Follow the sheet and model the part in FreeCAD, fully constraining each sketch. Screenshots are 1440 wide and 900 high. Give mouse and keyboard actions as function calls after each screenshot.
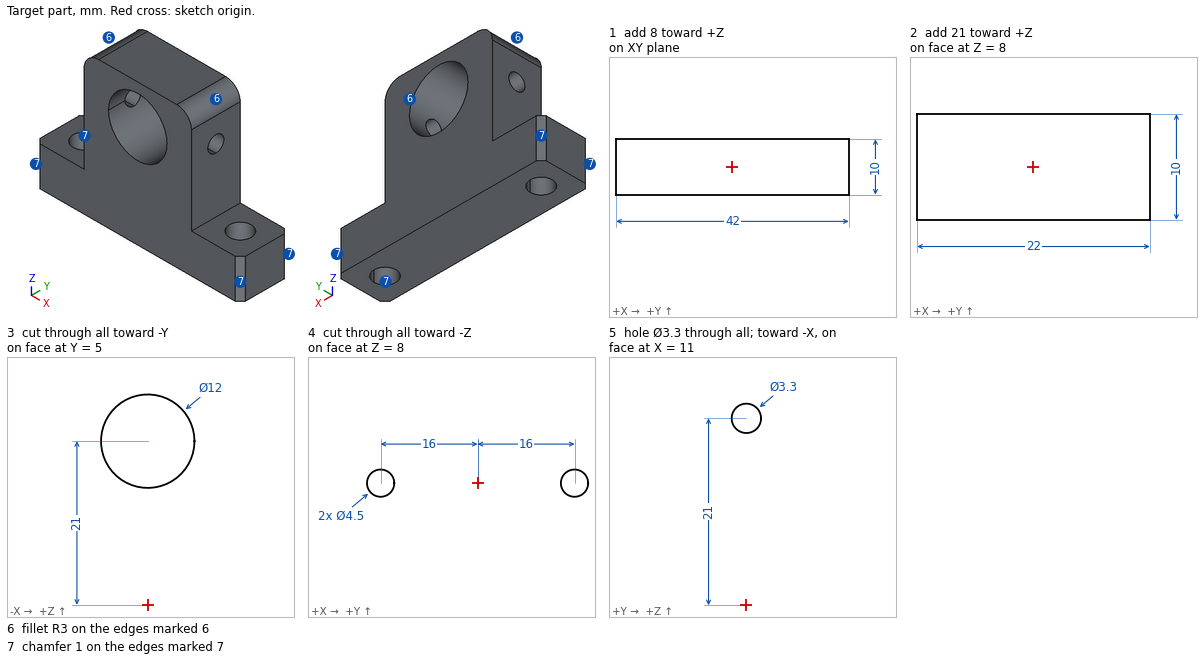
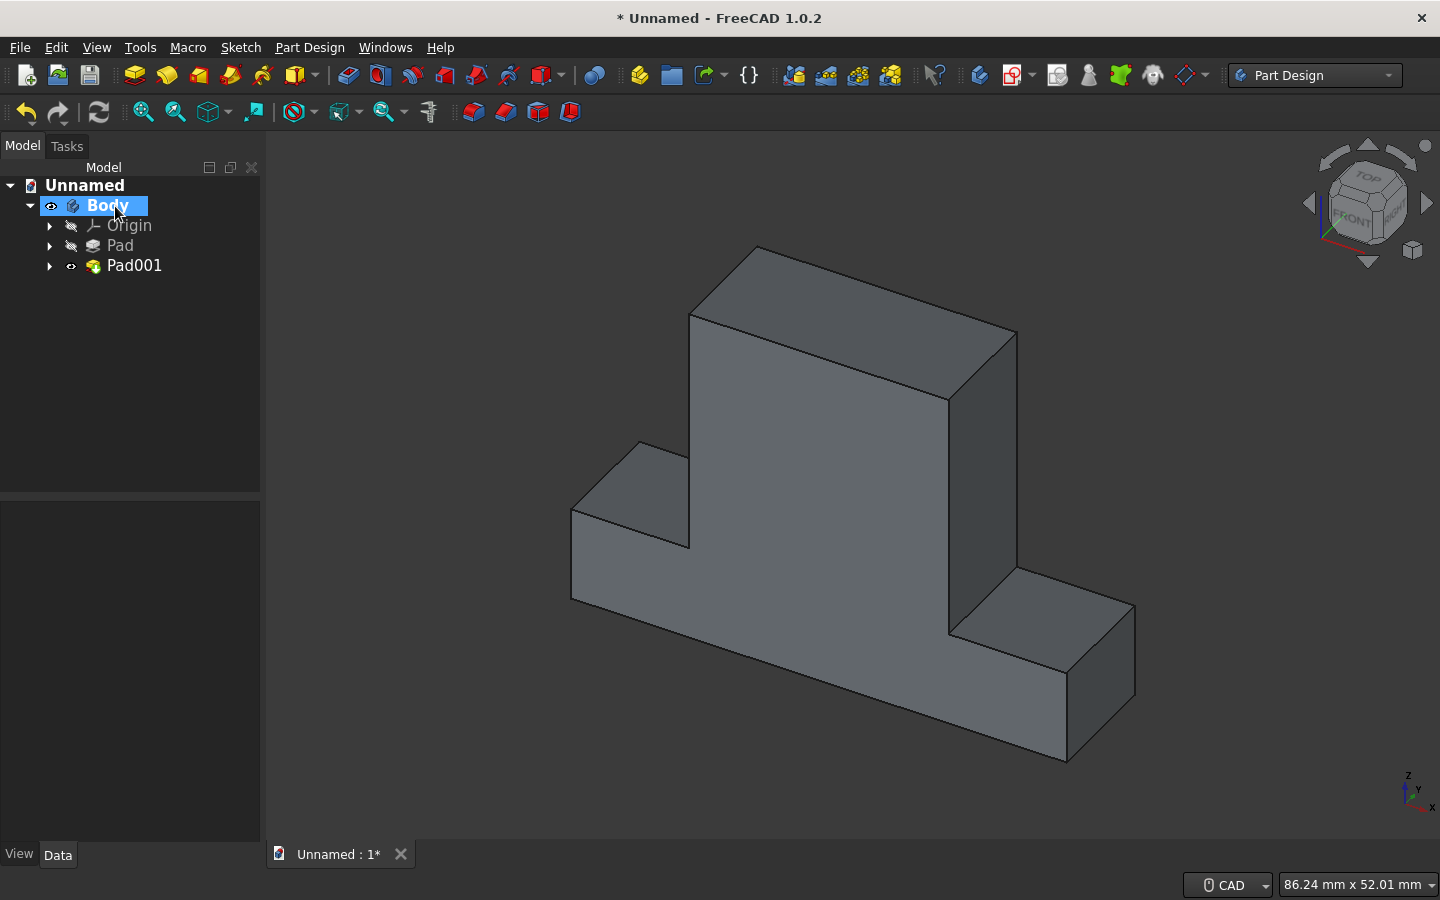
key(4)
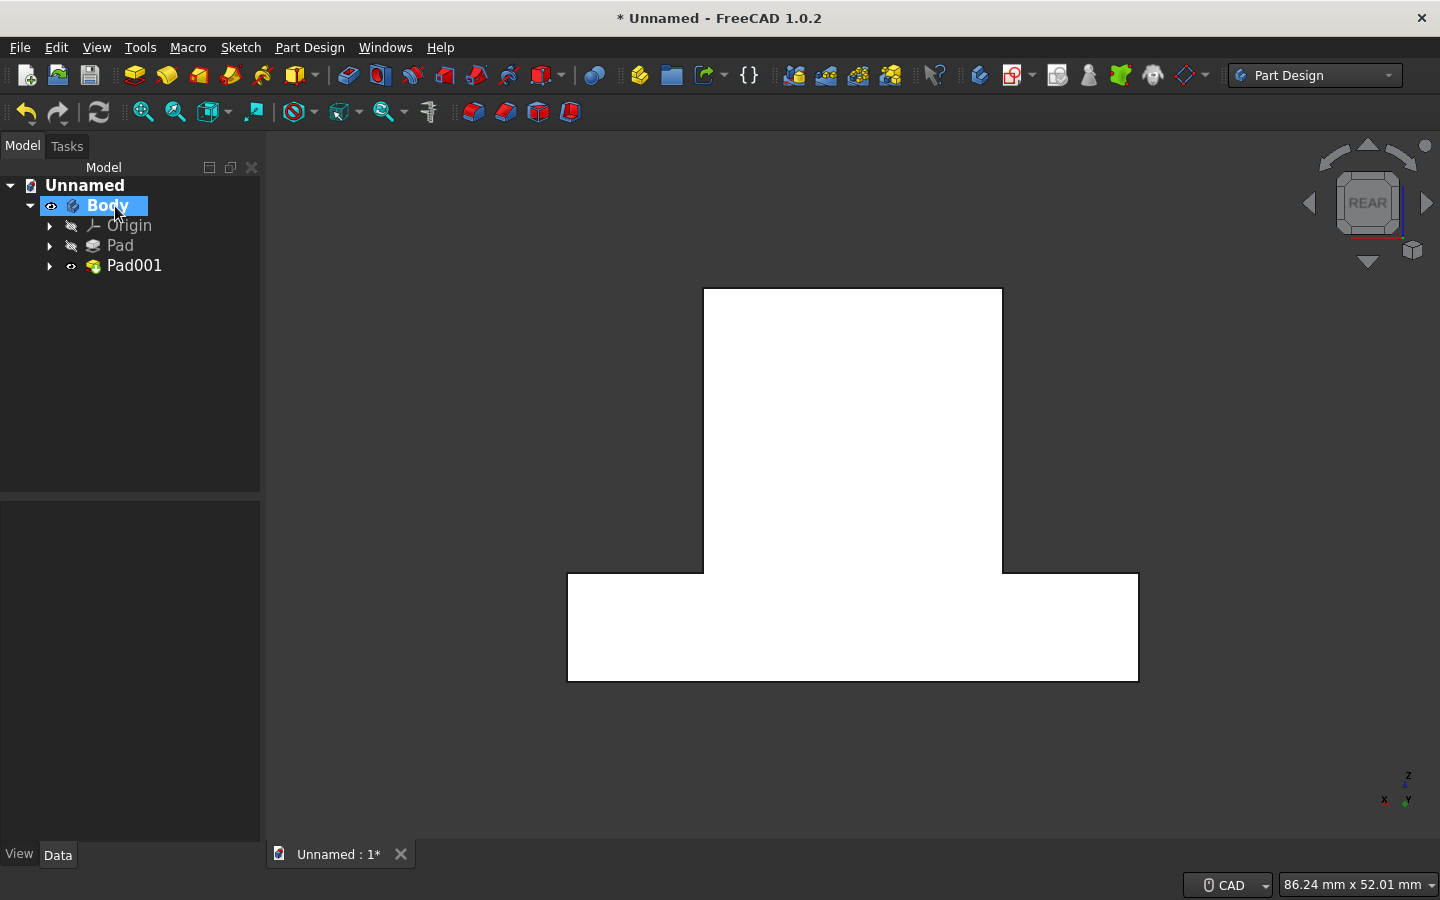
click(853, 484)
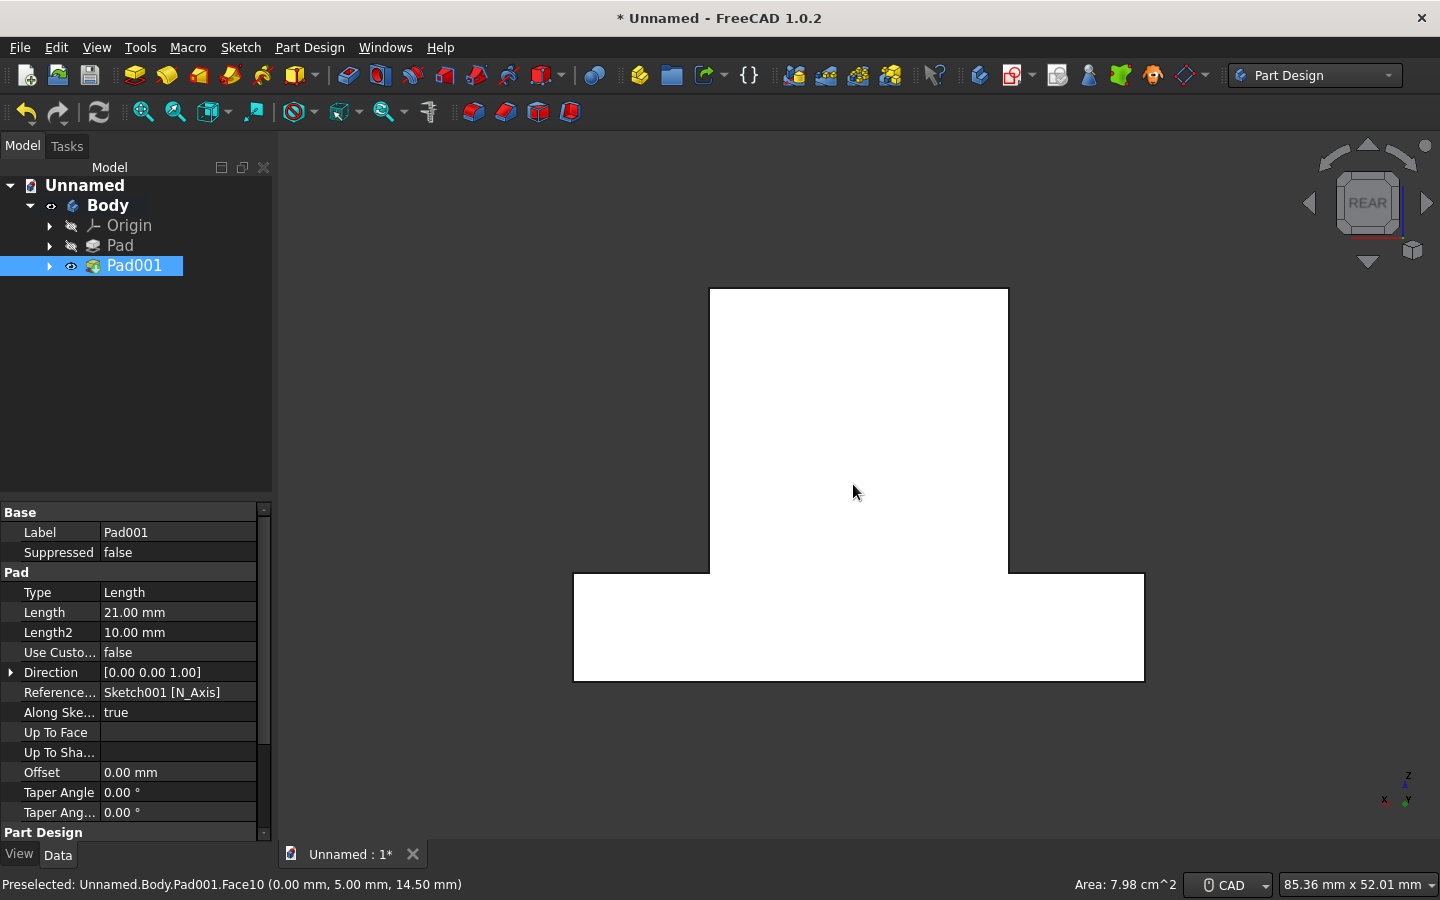
click(1012, 76)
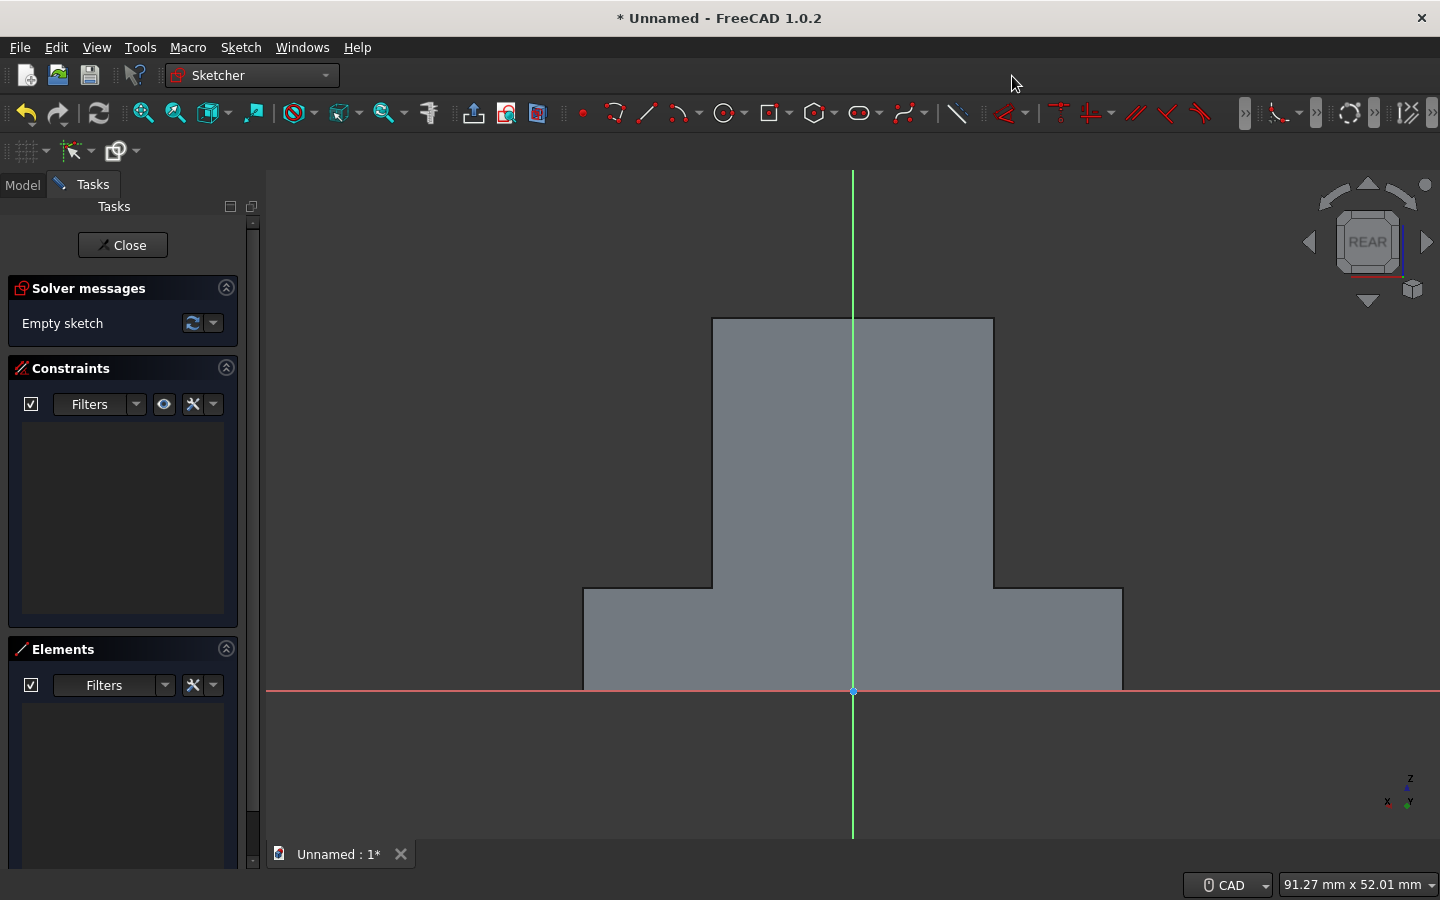
click(724, 114)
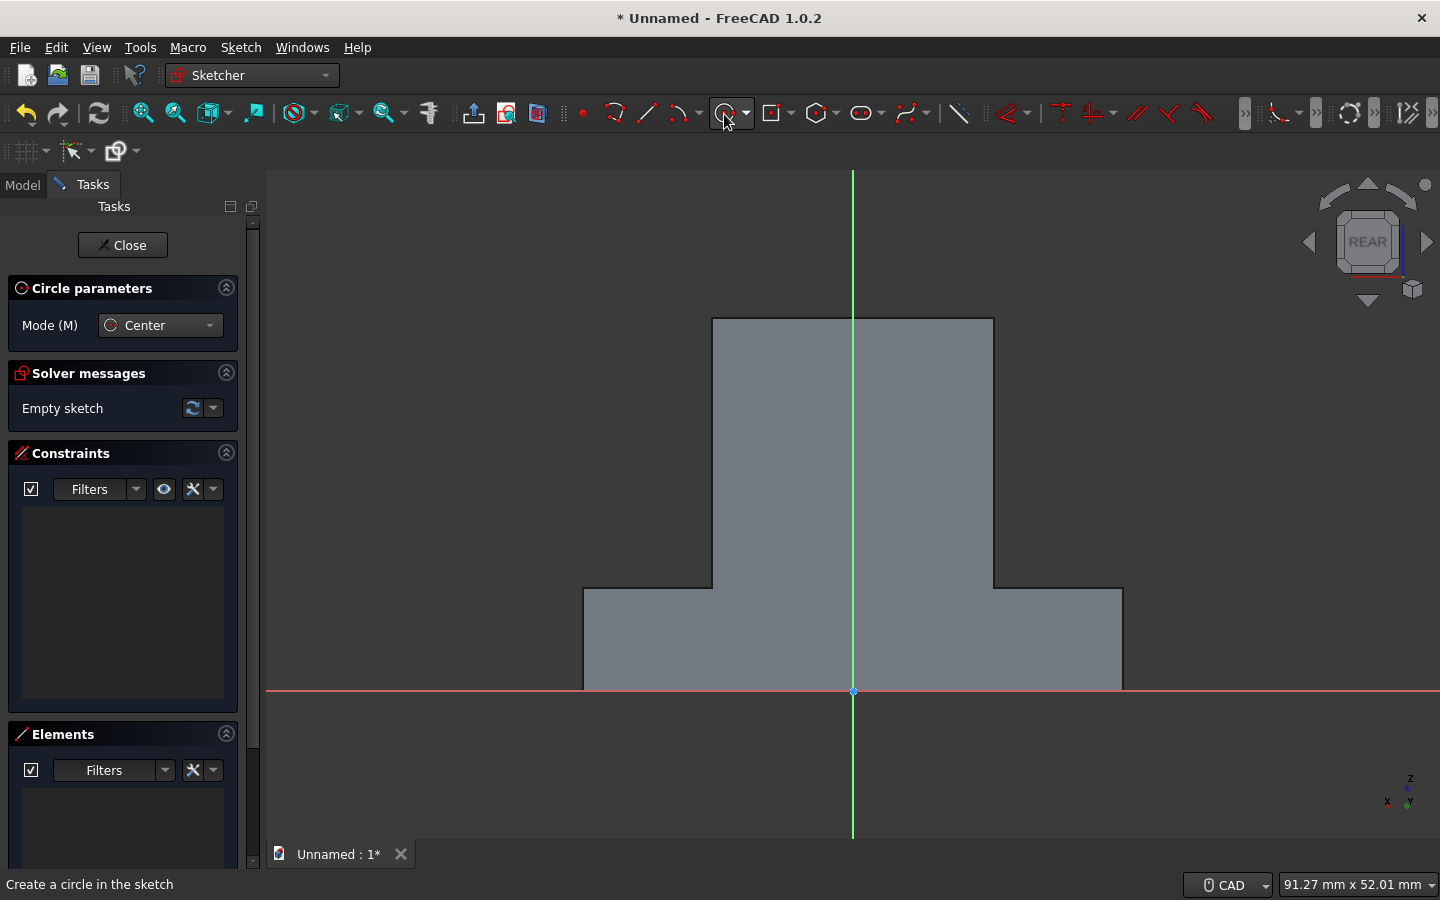
click(853, 421)
click(908, 366)
key(Escape)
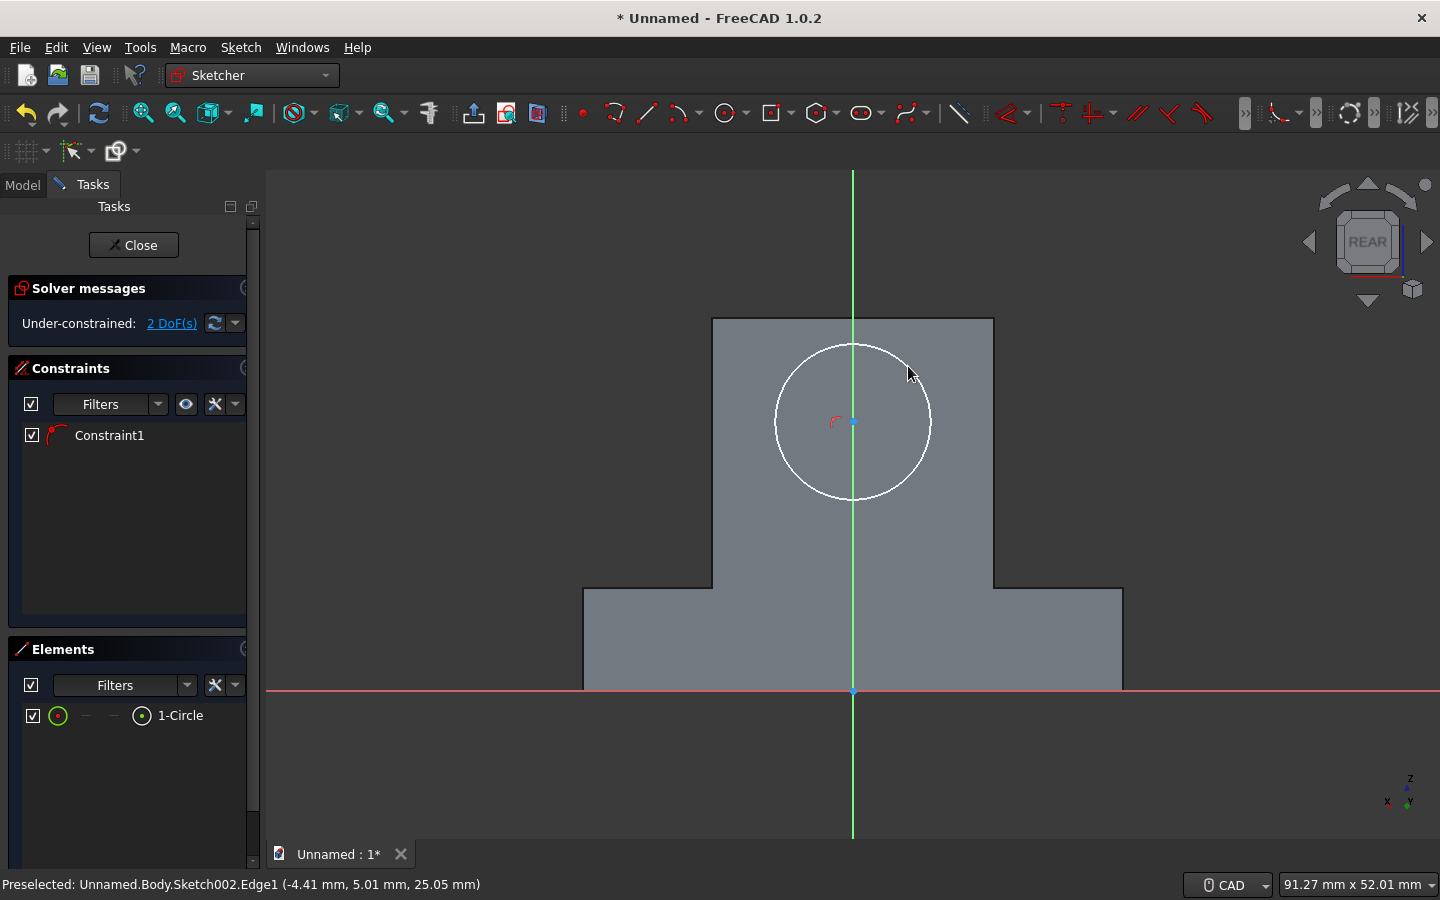
click(1006, 114)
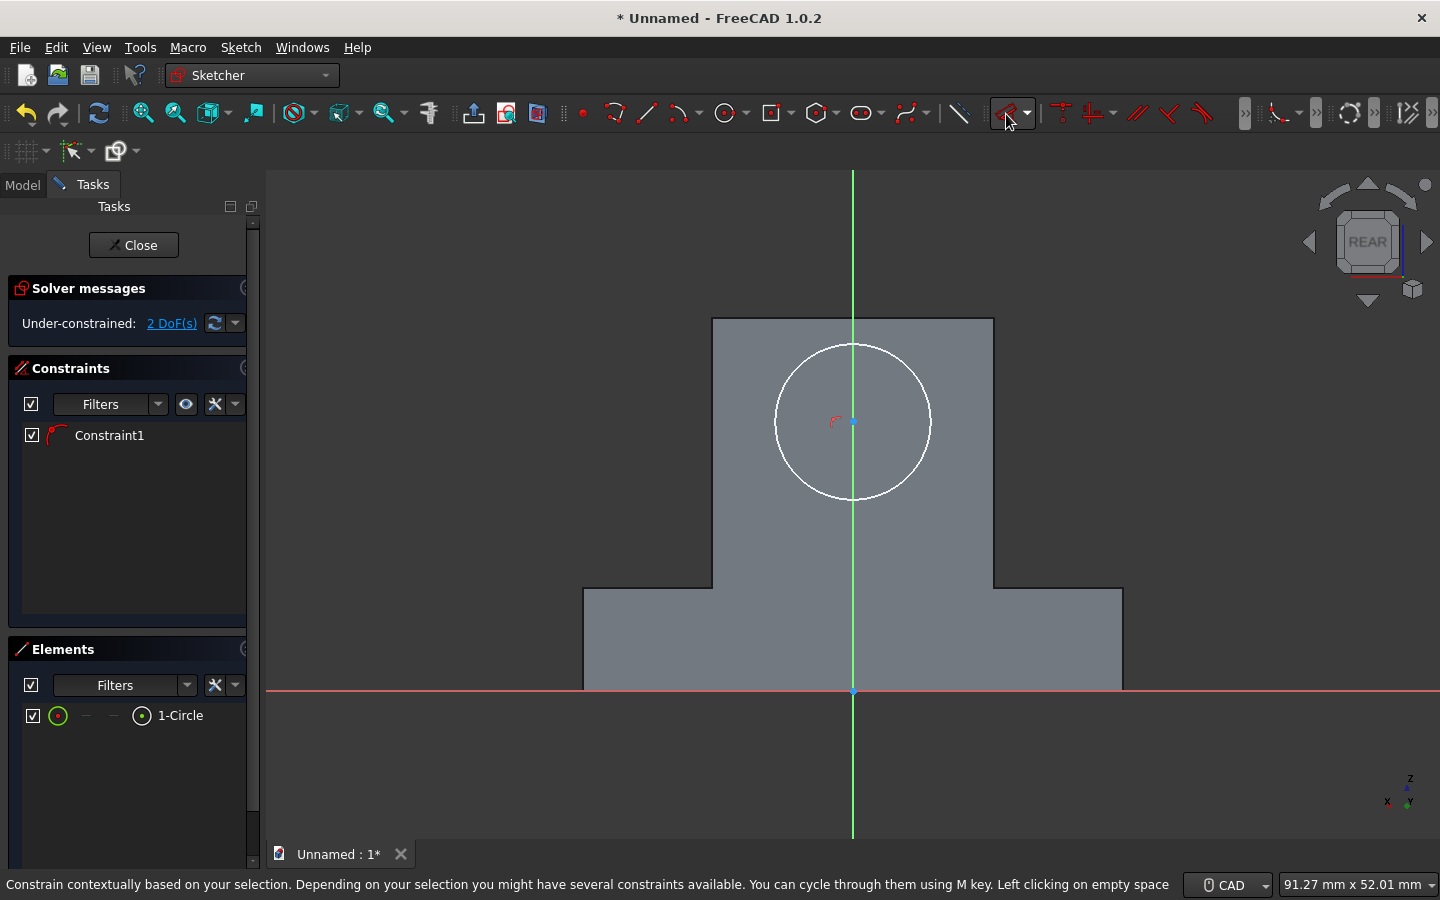
click(908, 367)
click(931, 344)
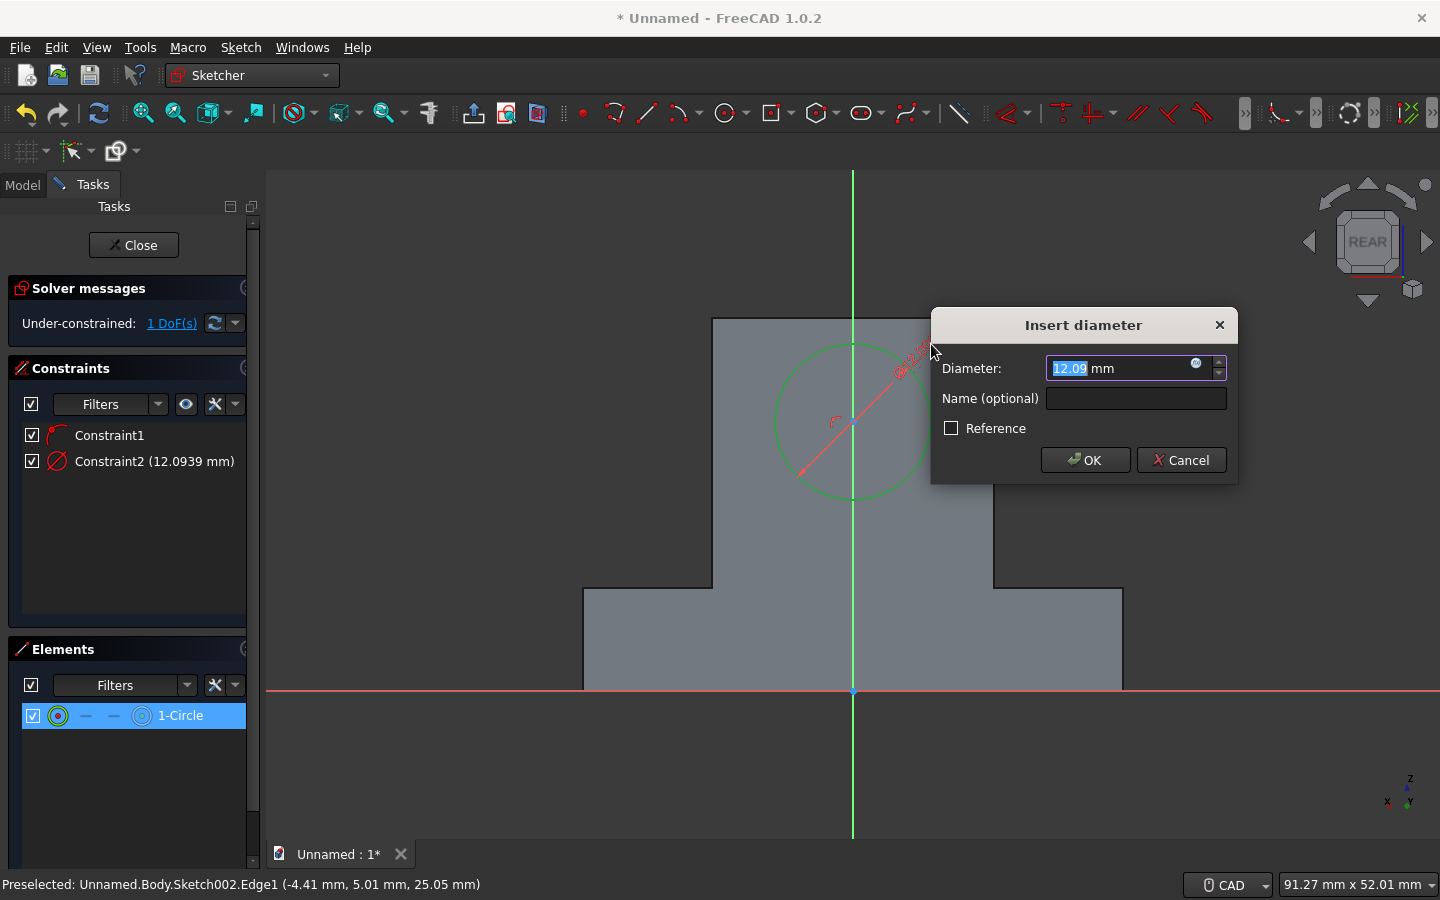
text(12)
key(Return)